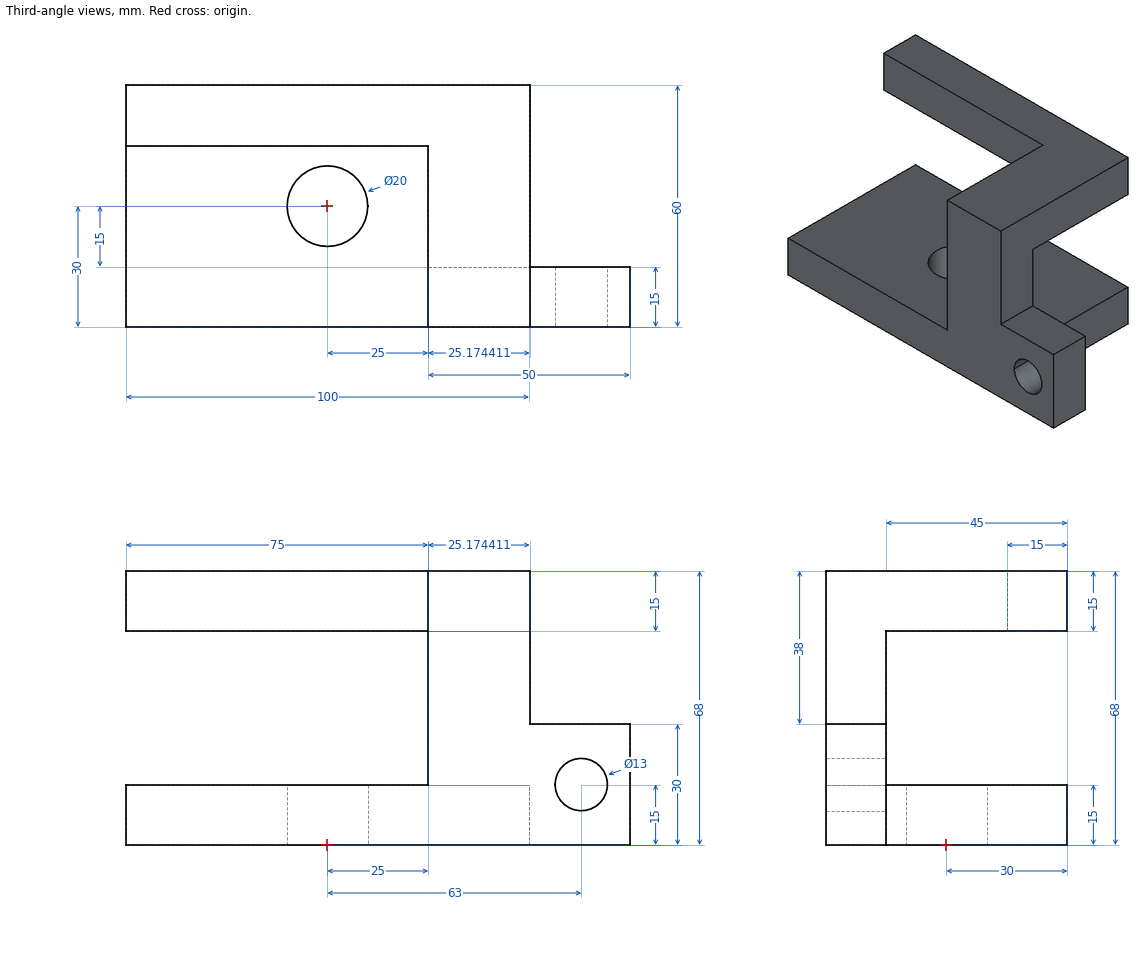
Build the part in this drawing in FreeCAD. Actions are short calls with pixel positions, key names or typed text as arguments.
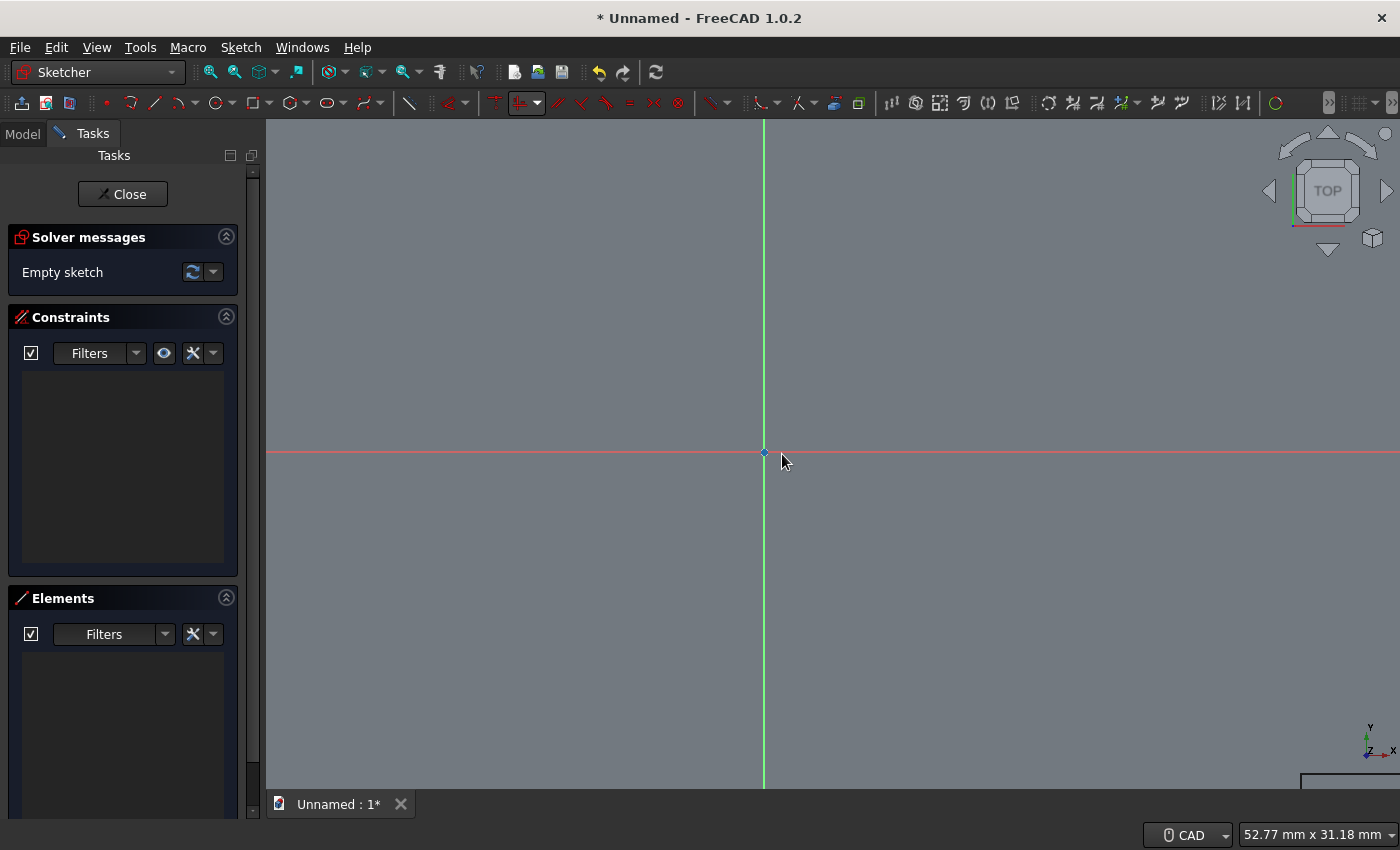
click(216, 104)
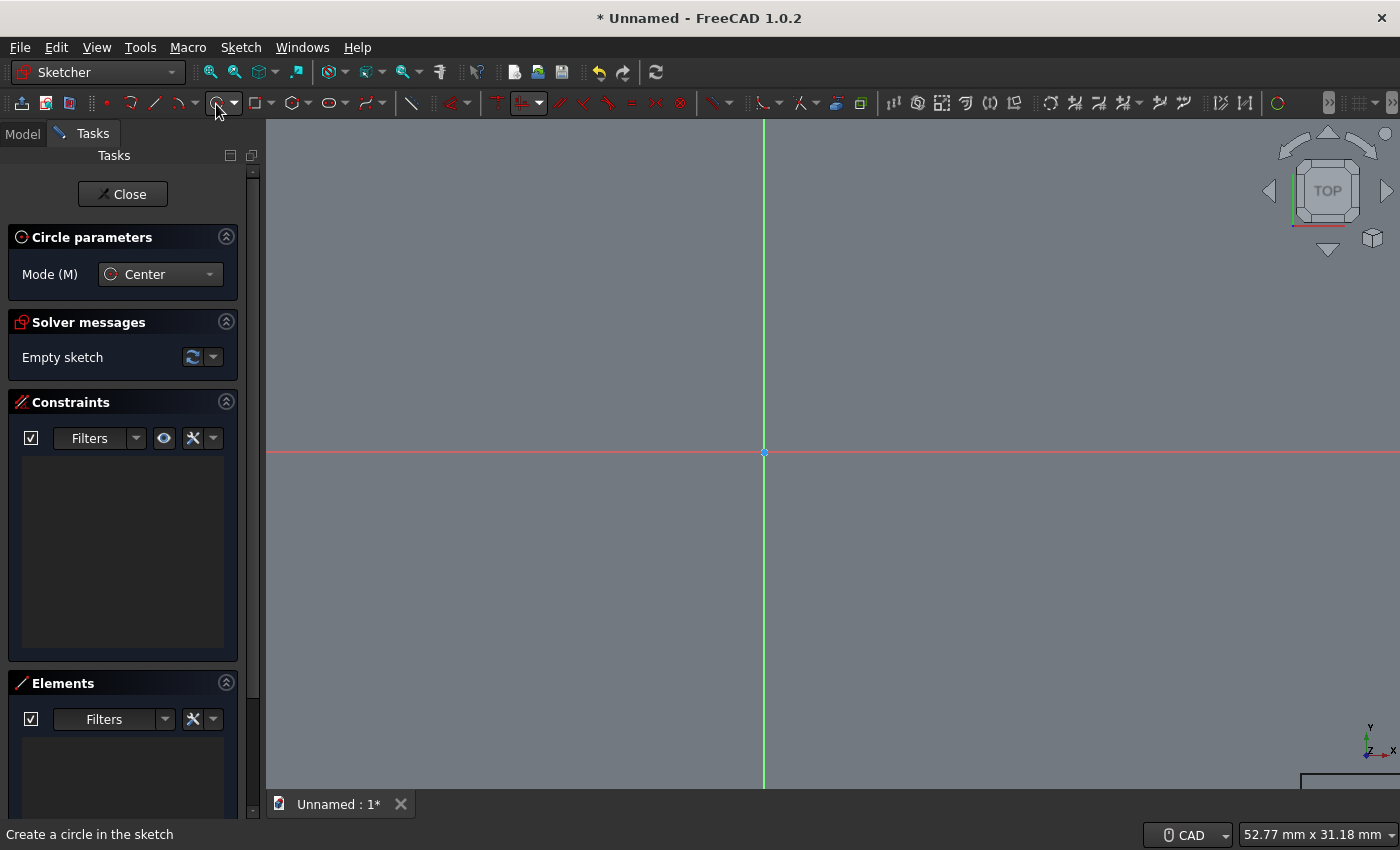
click(764, 452)
move(916, 300)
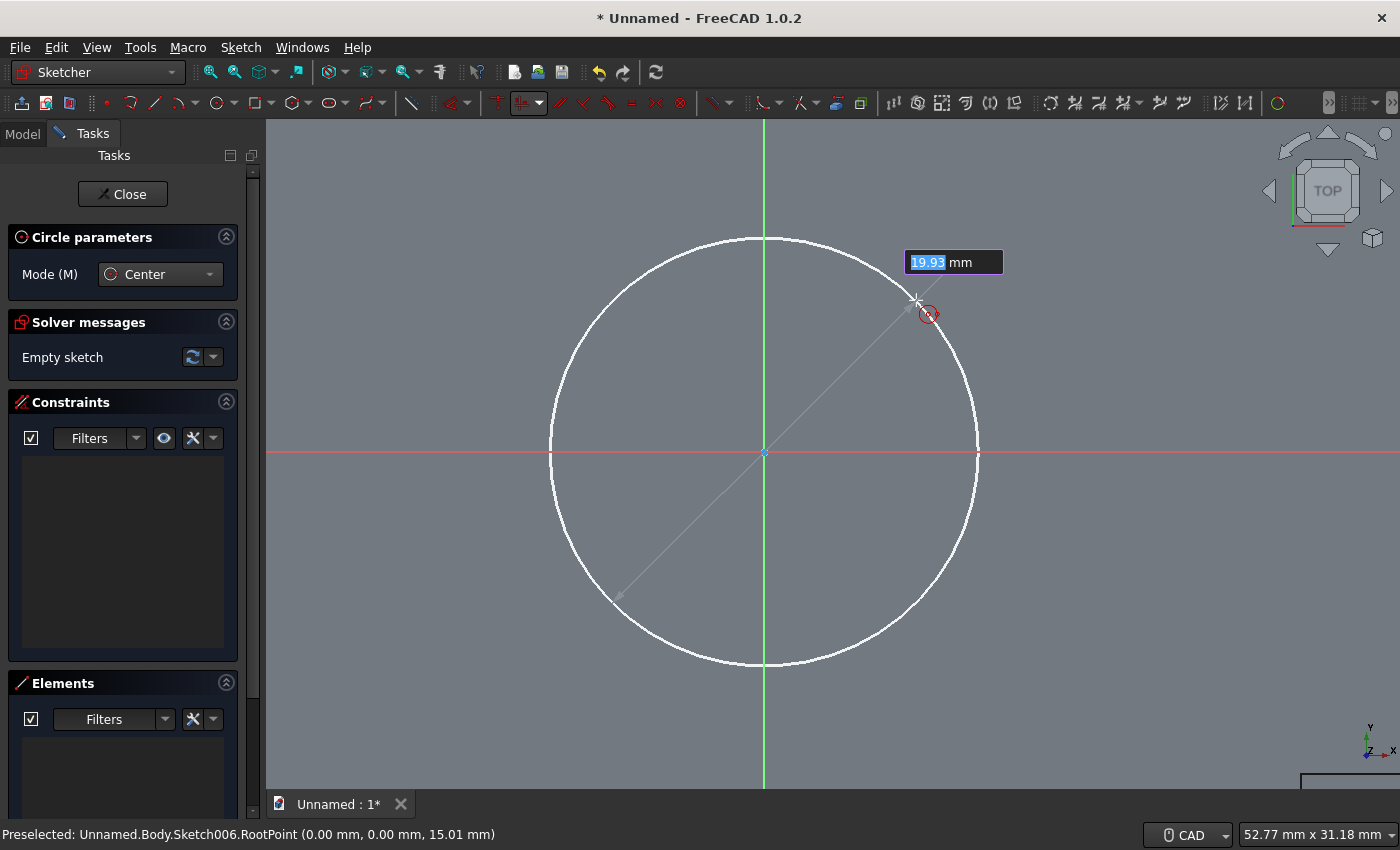
text(20)
key(Return)
key(Escape)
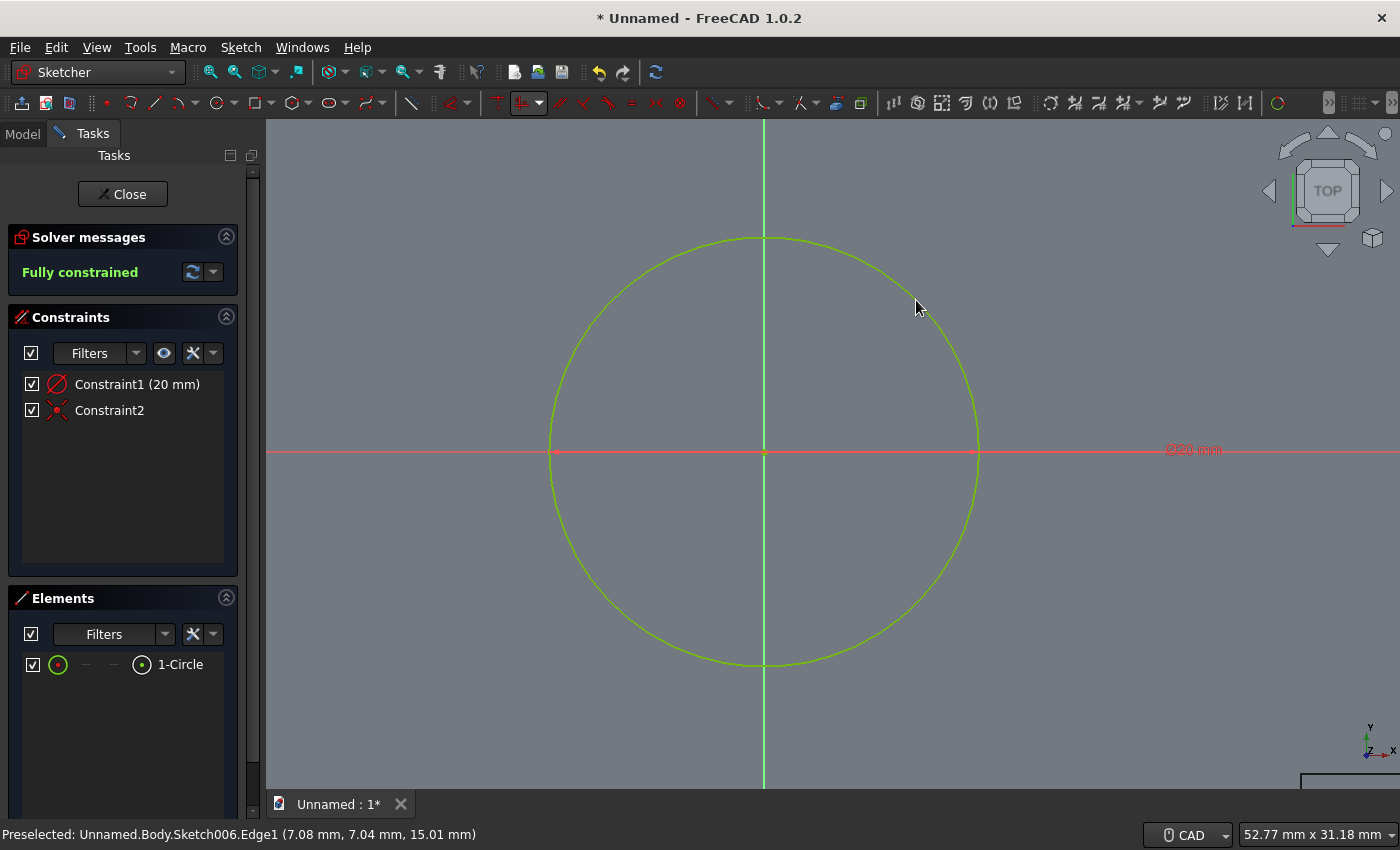
click(123, 194)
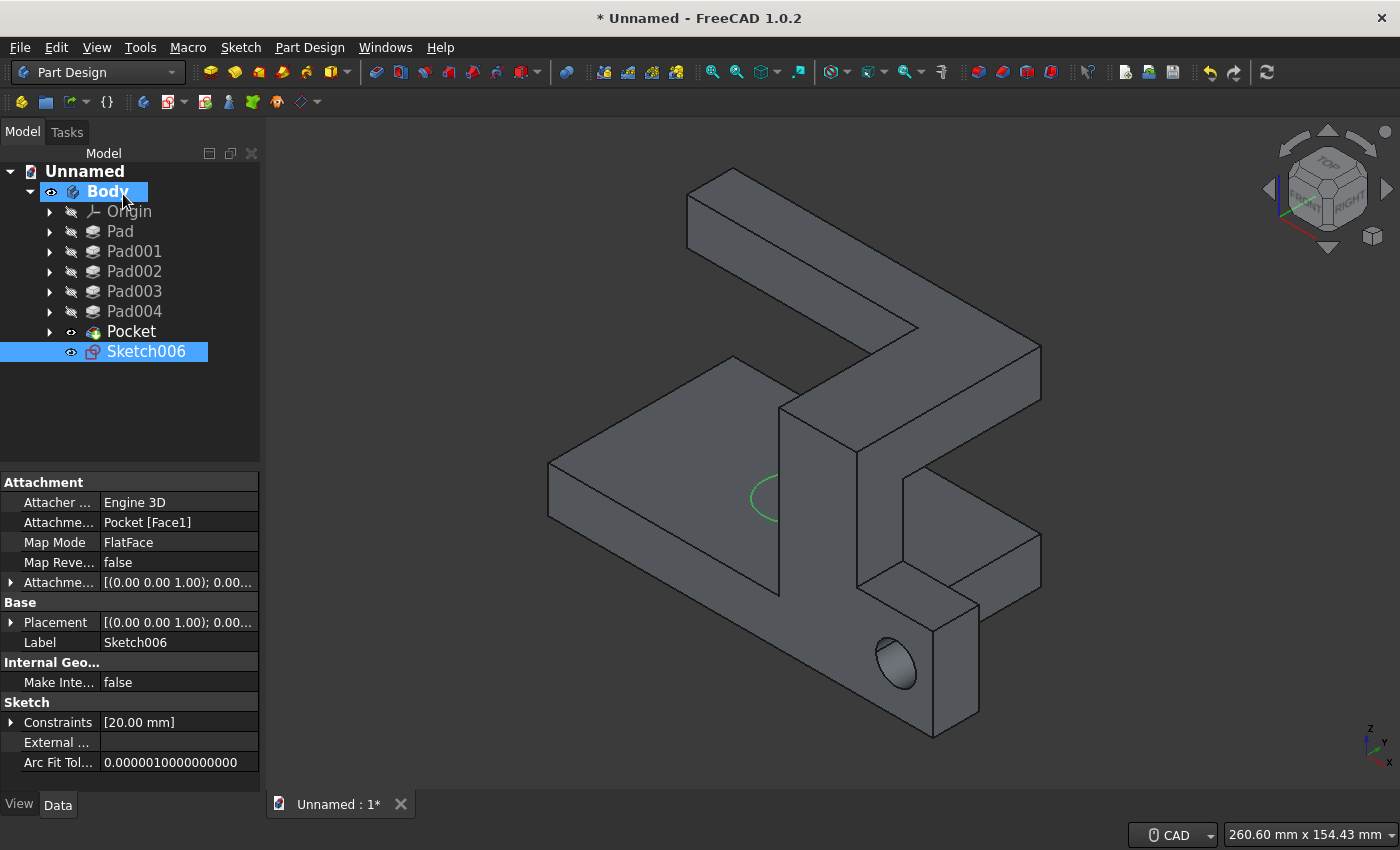
click(378, 72)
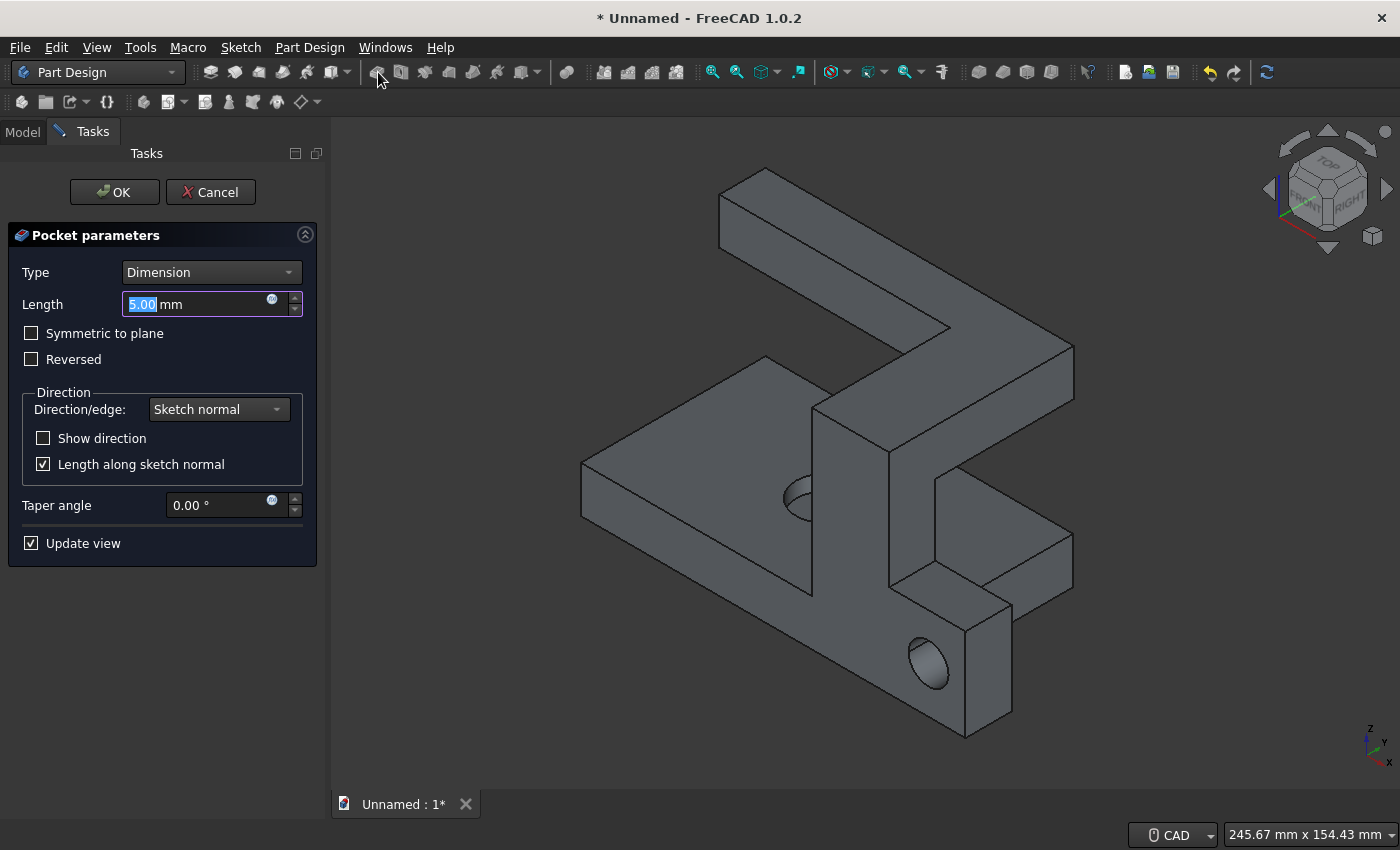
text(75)
key(Tab)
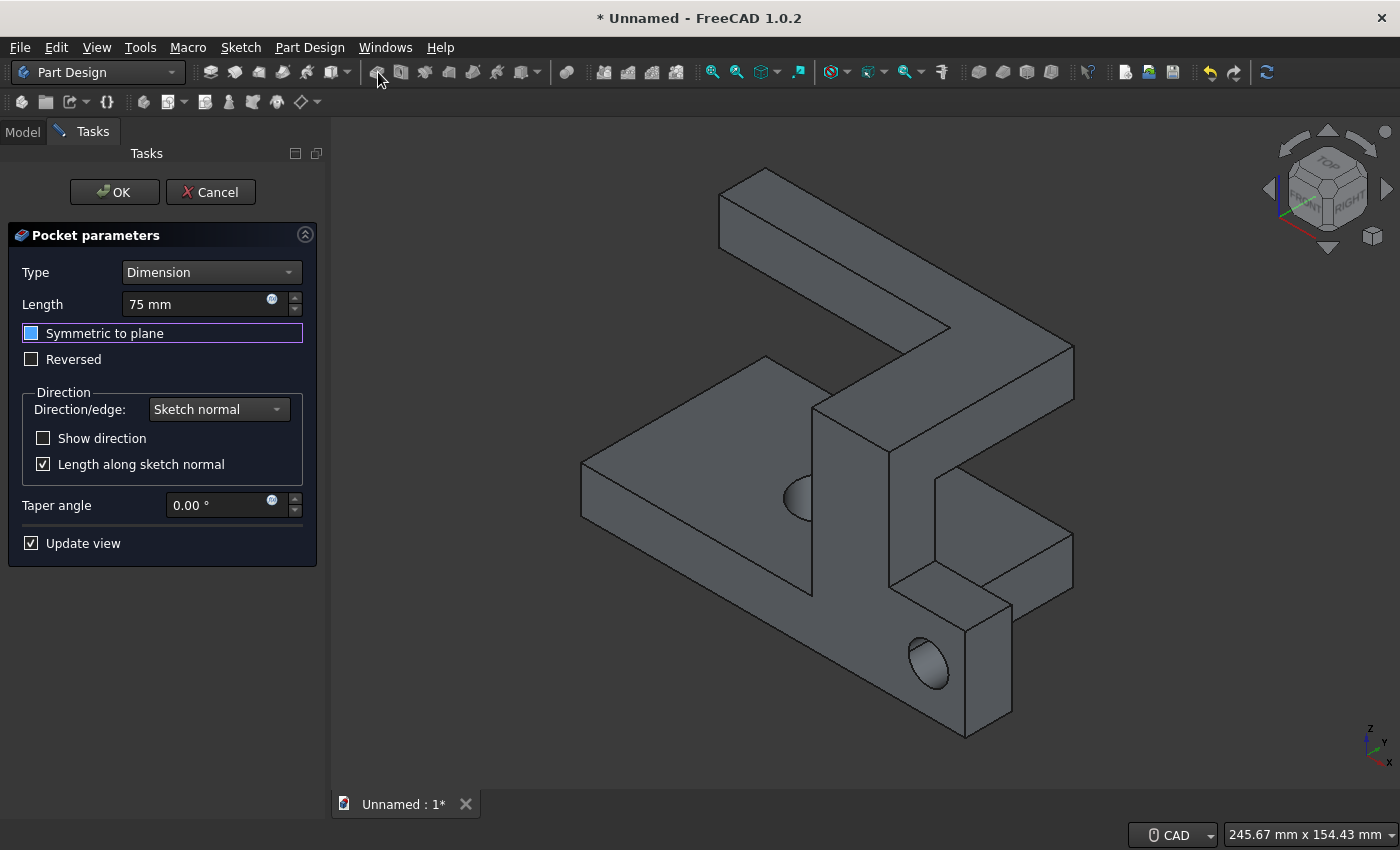
click(115, 192)